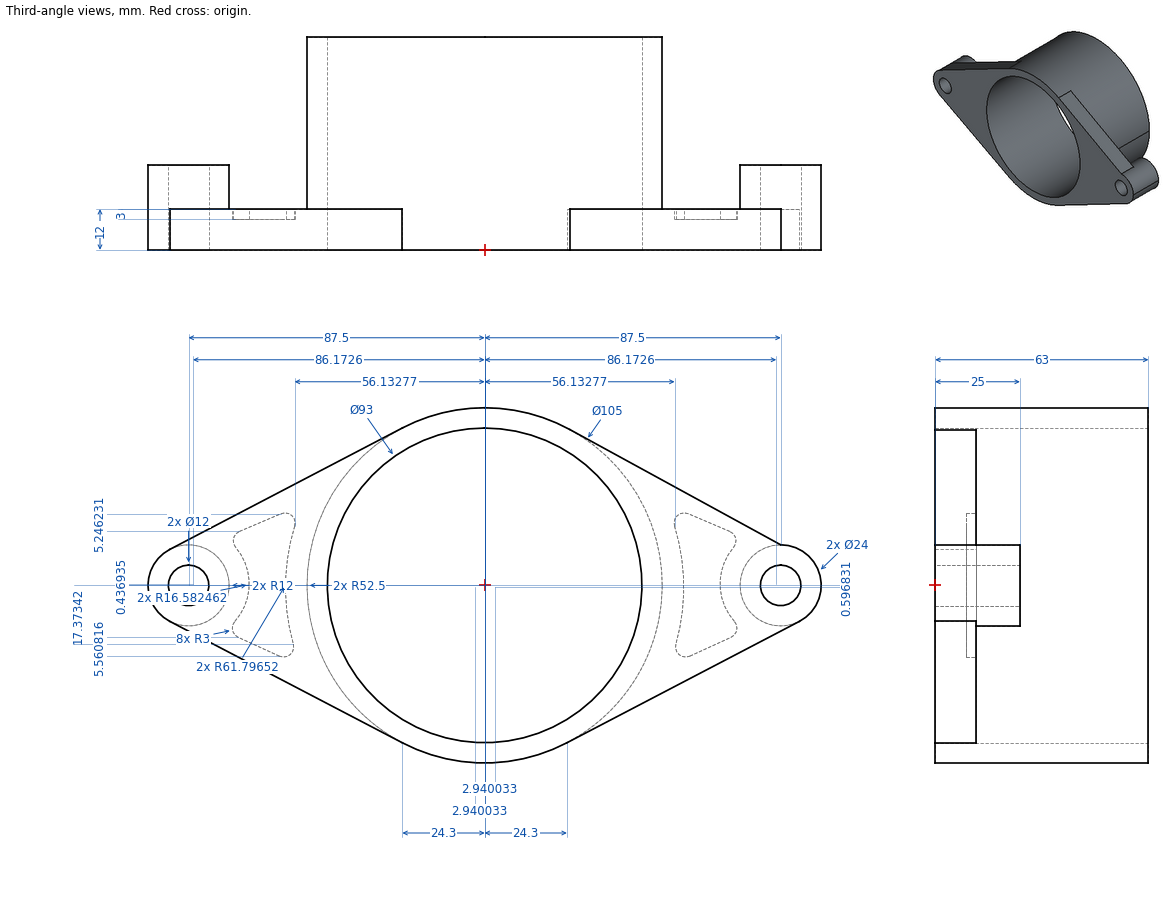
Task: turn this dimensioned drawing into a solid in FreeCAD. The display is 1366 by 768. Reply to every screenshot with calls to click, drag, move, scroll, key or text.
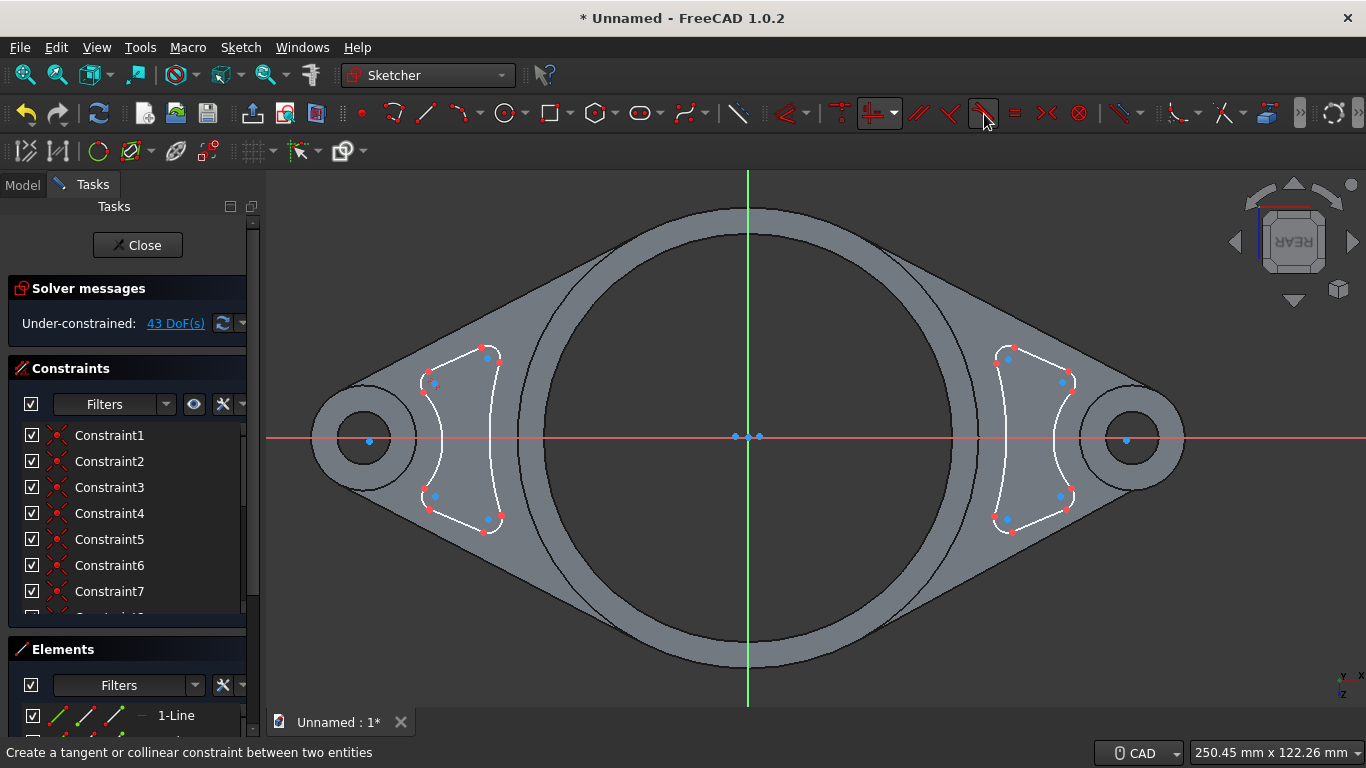
click(466, 355)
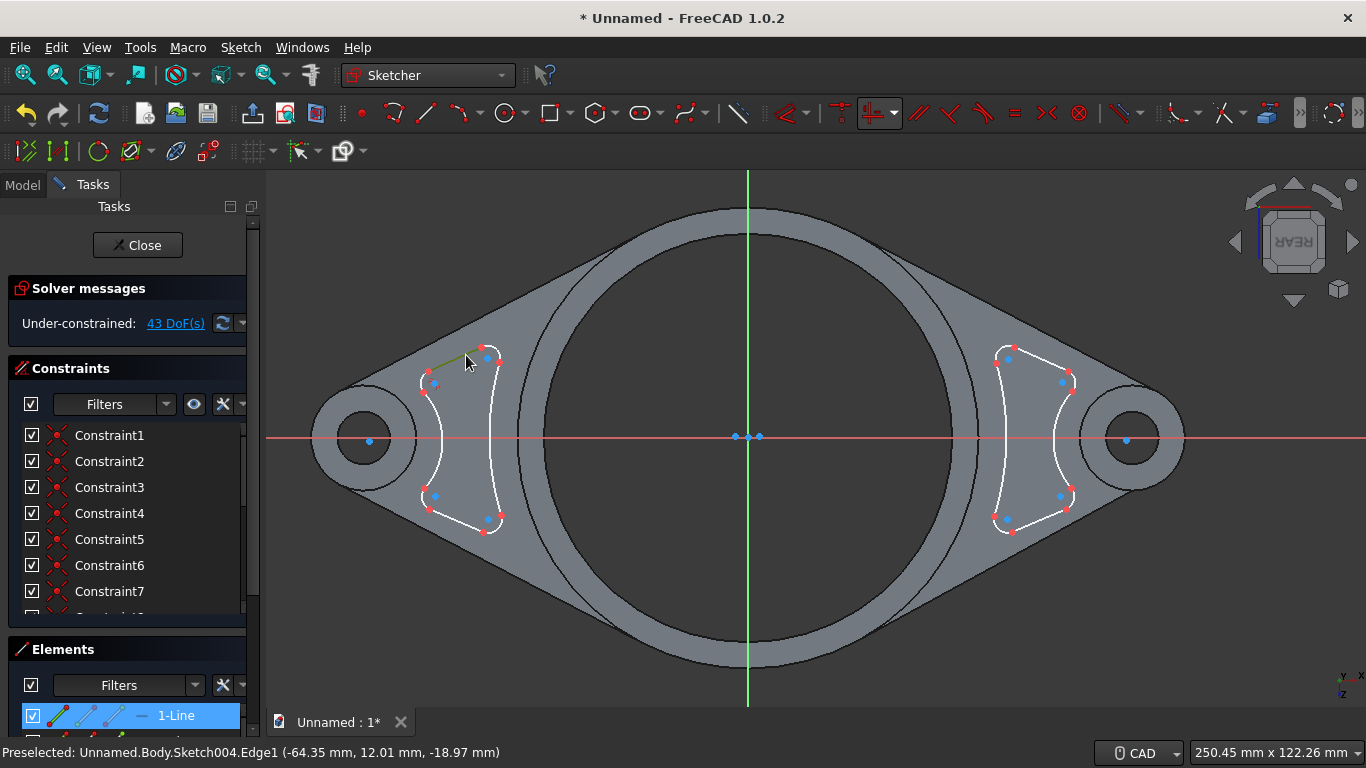
click(496, 349)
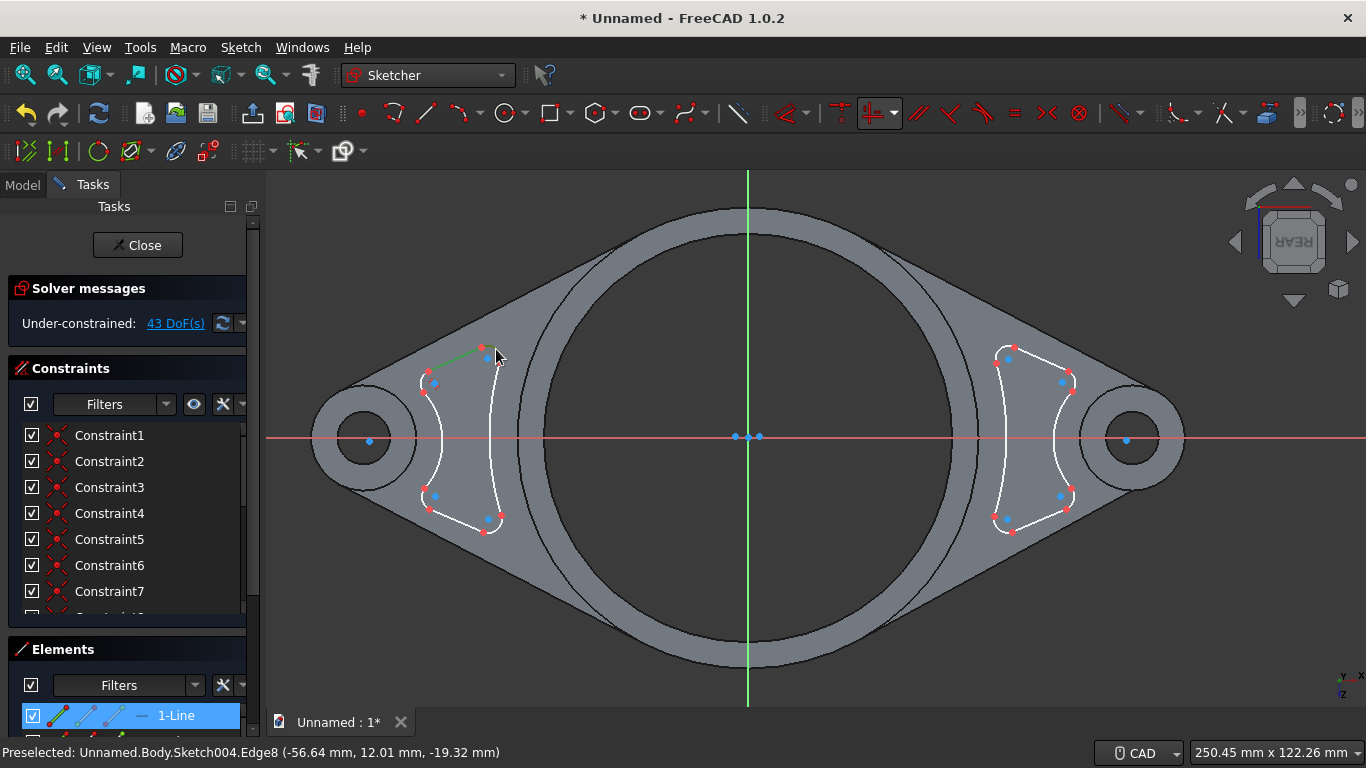
click(984, 114)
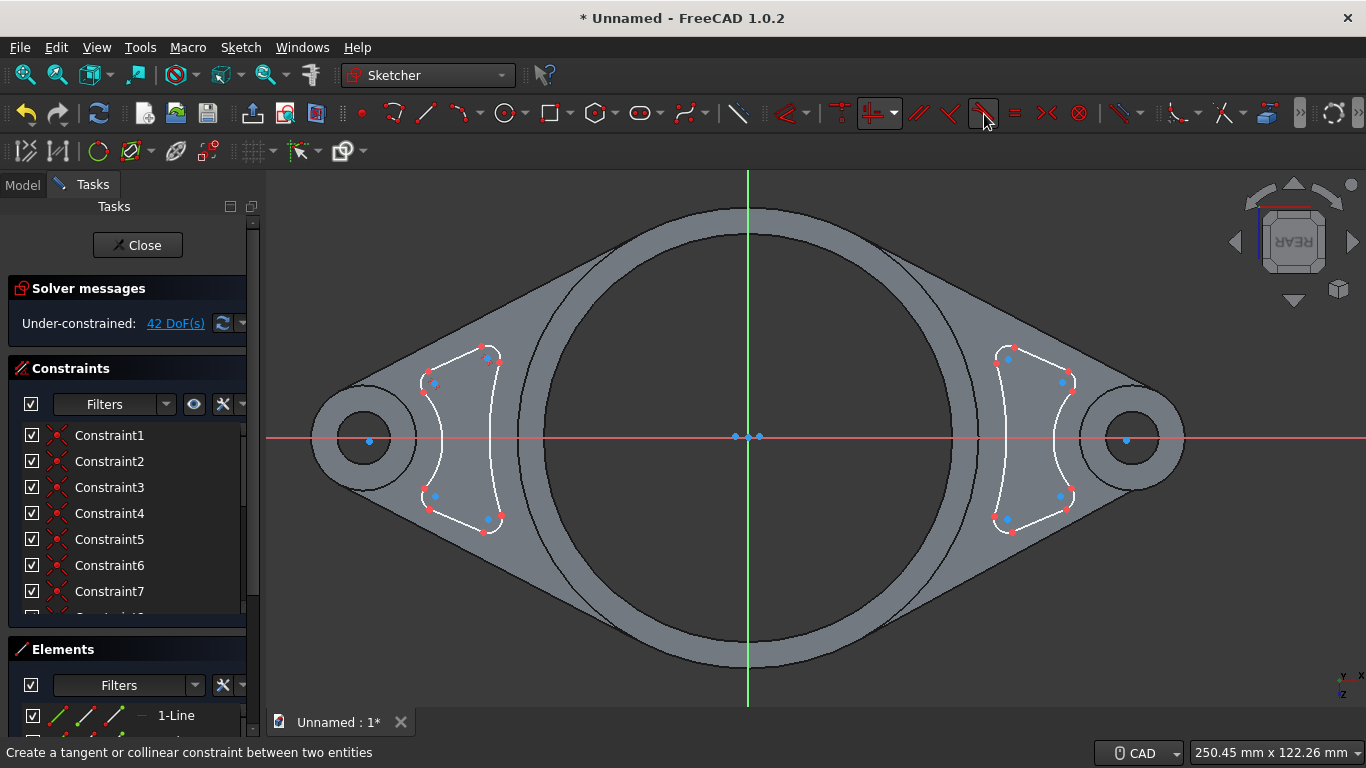
click(446, 516)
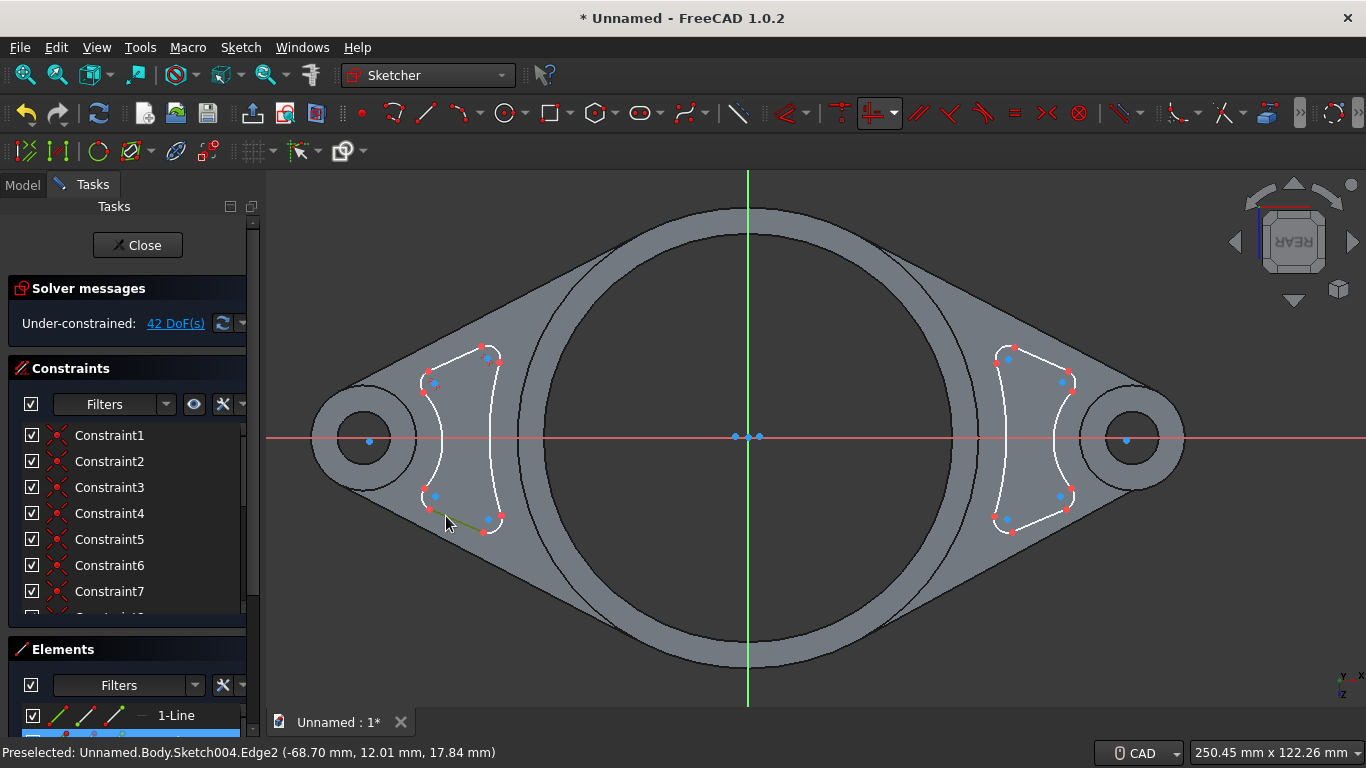
click(422, 500)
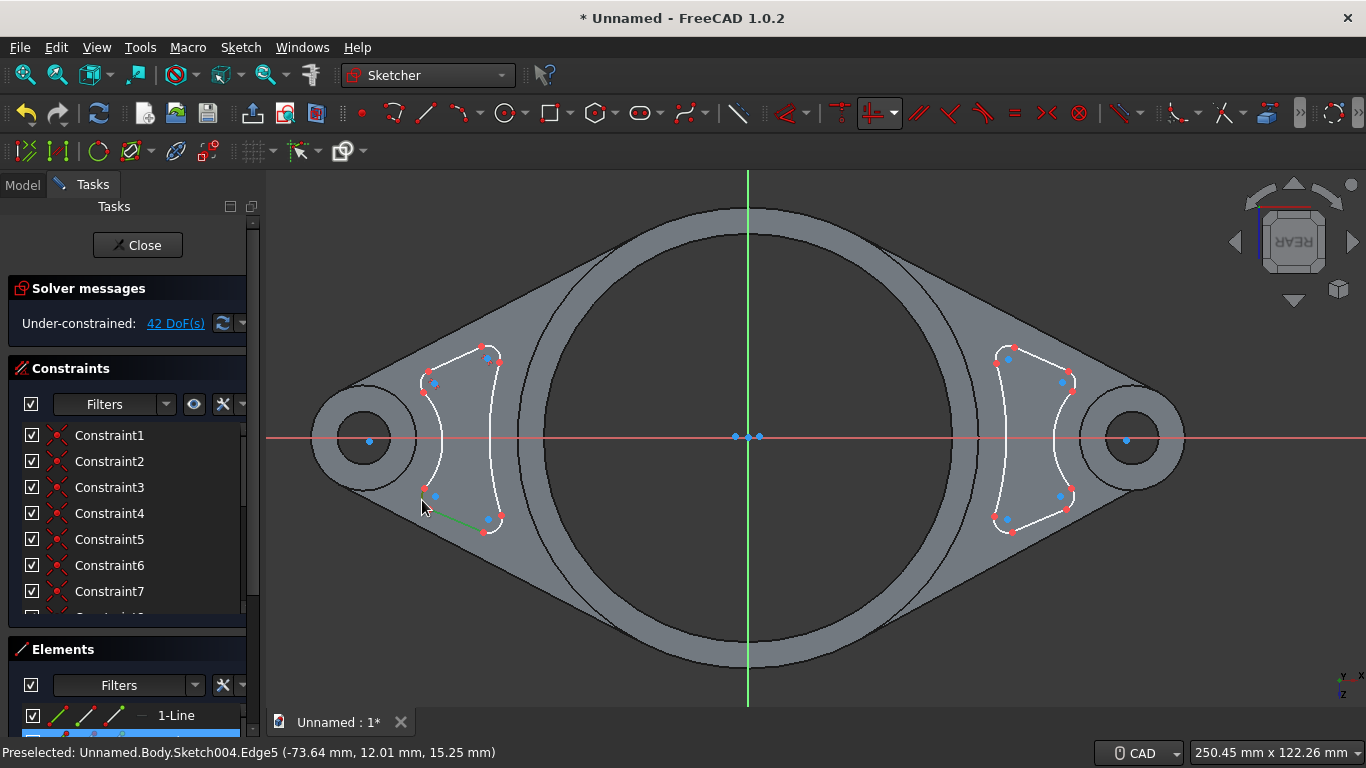
key(t)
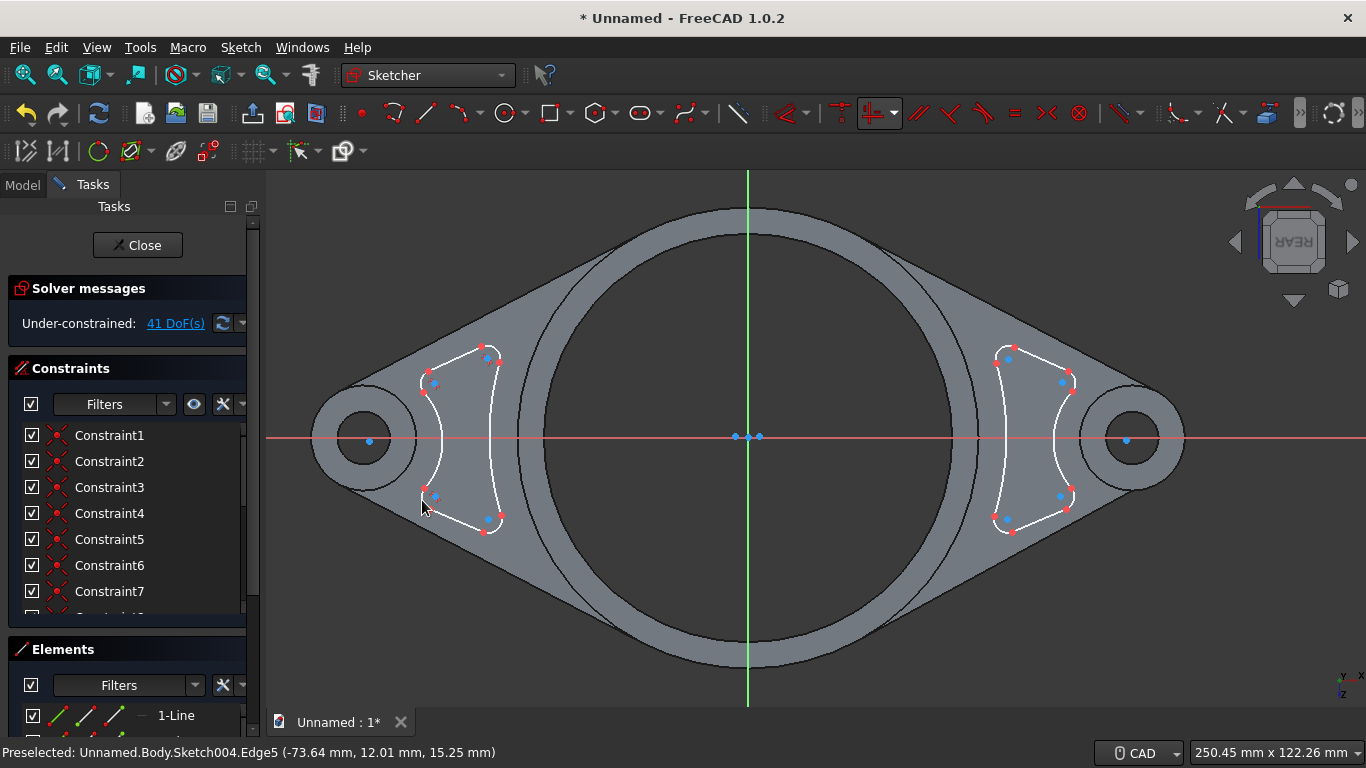
click(446, 516)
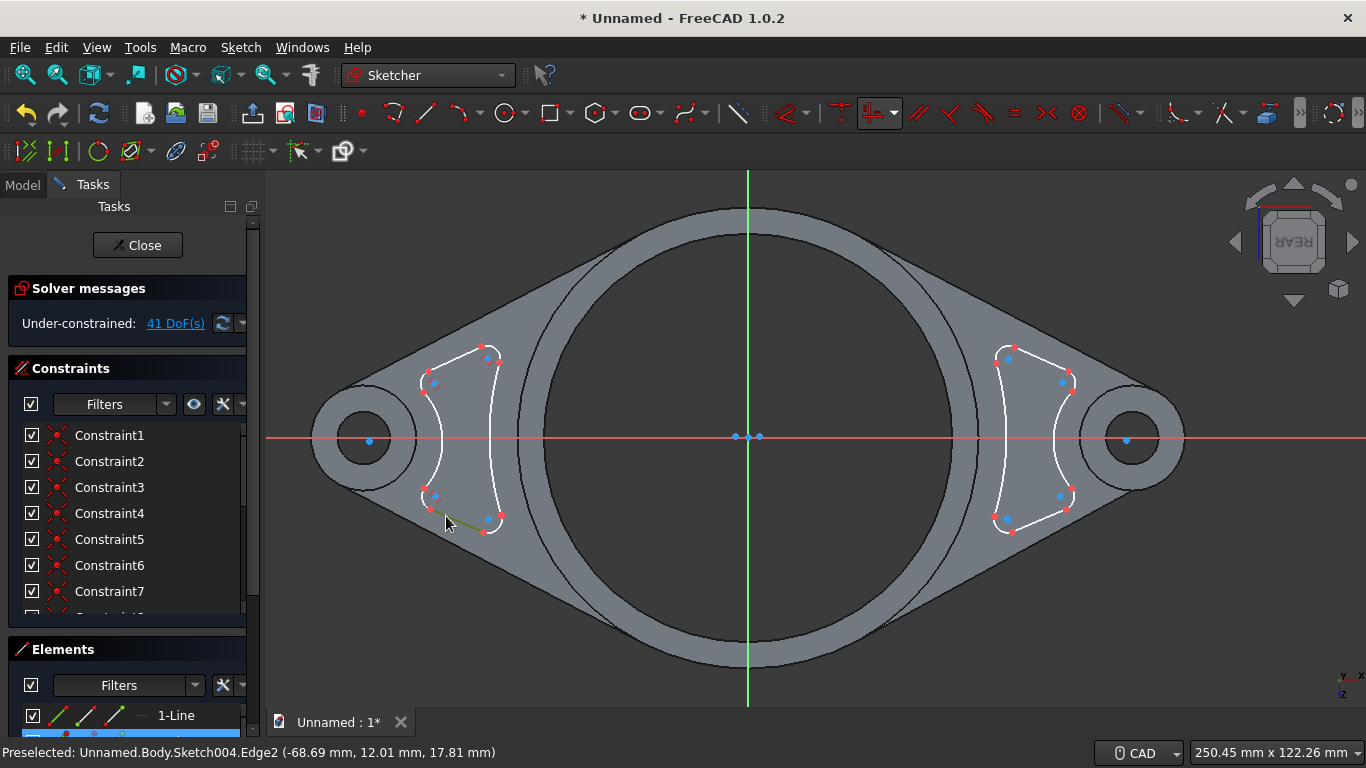
click(498, 529)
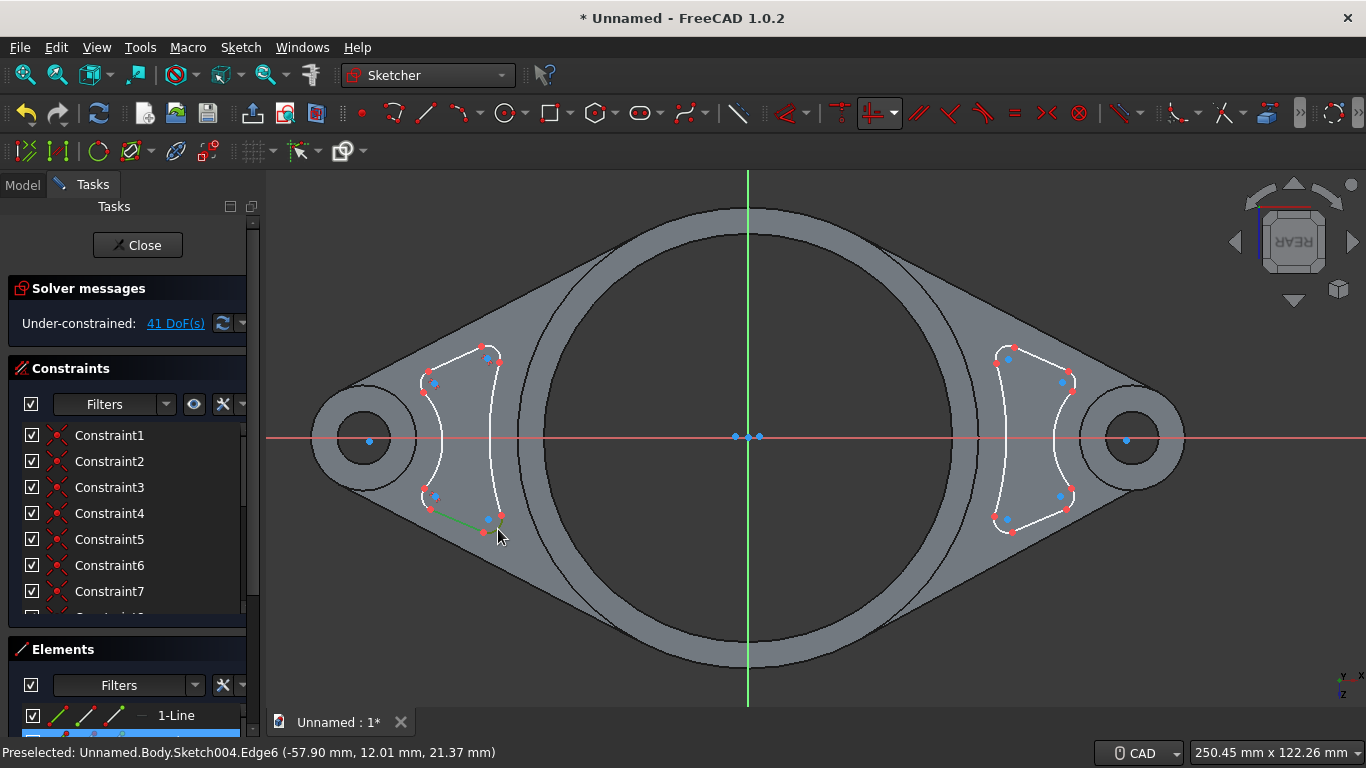
click(984, 114)